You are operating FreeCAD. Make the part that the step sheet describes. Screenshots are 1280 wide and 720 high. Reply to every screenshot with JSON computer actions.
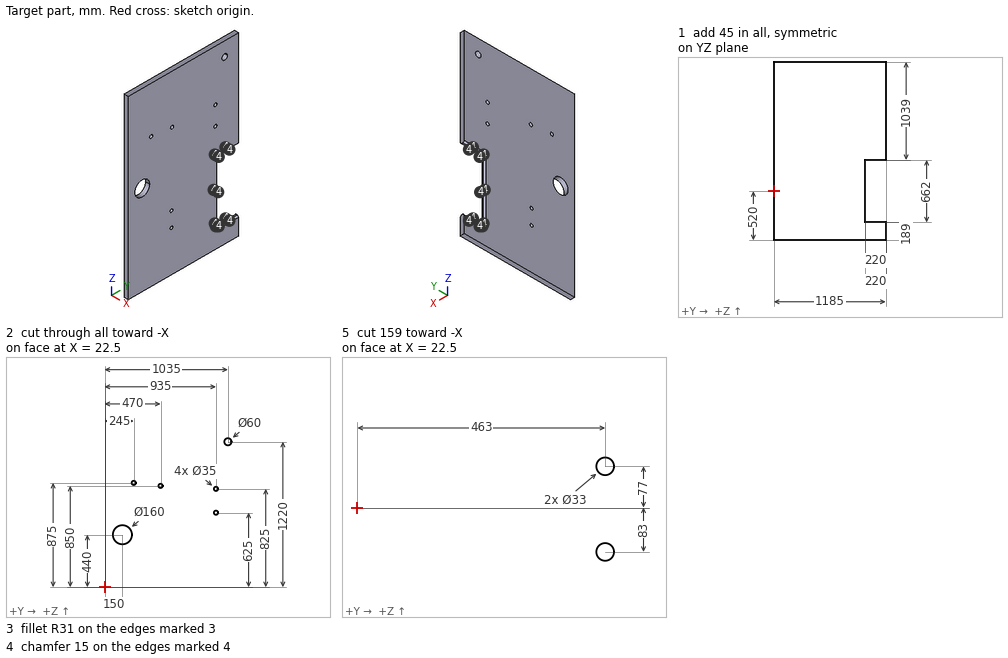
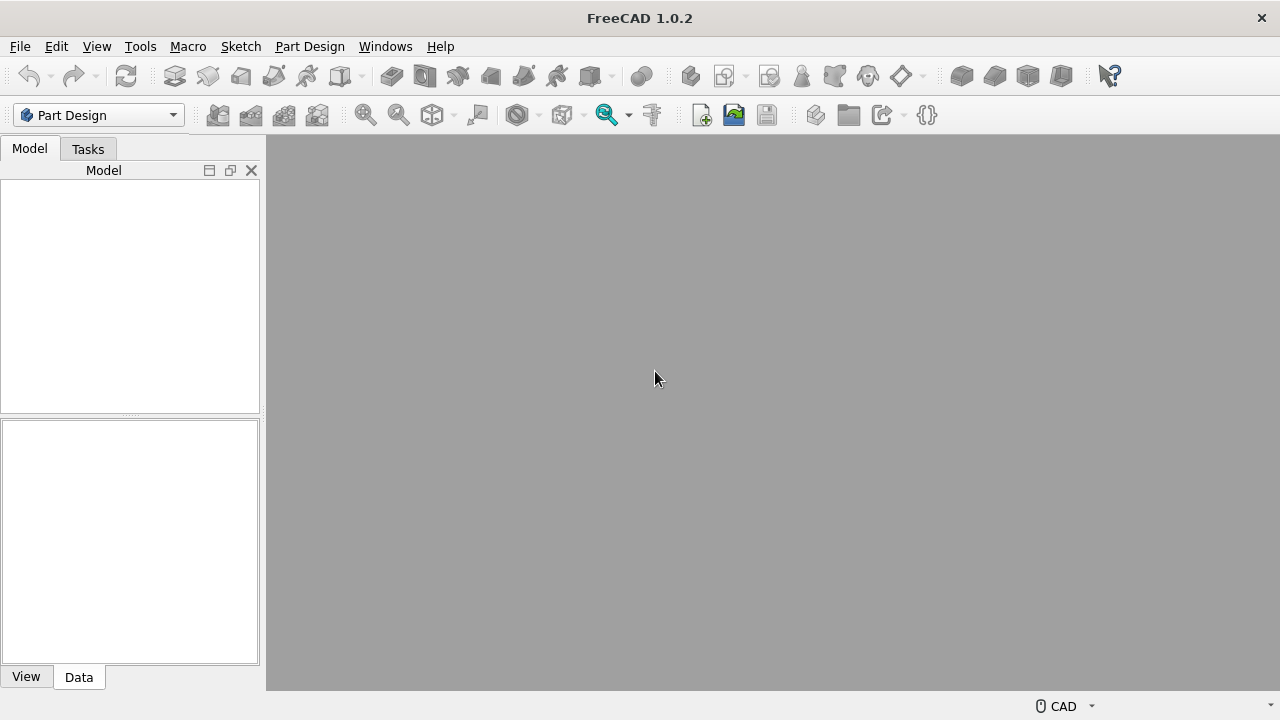
{"action": "left_click", "coordinate": [701, 116]}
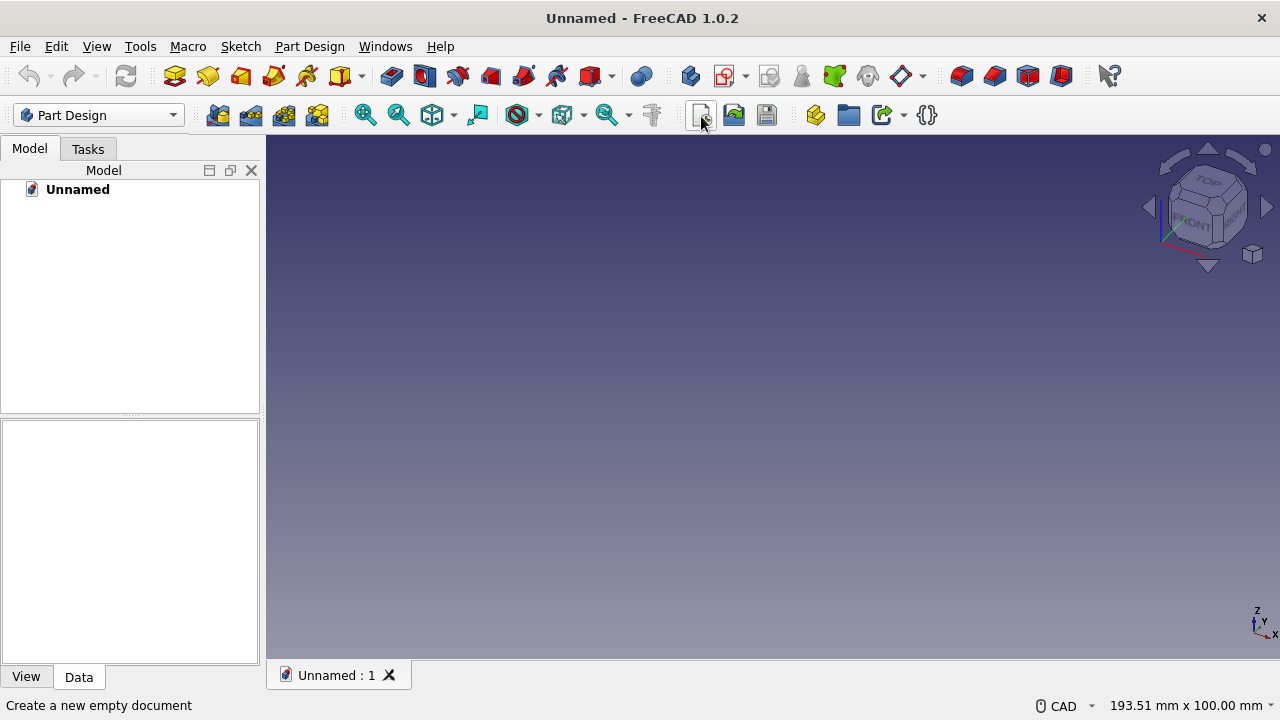
{"action": "left_click", "coordinate": [724, 76]}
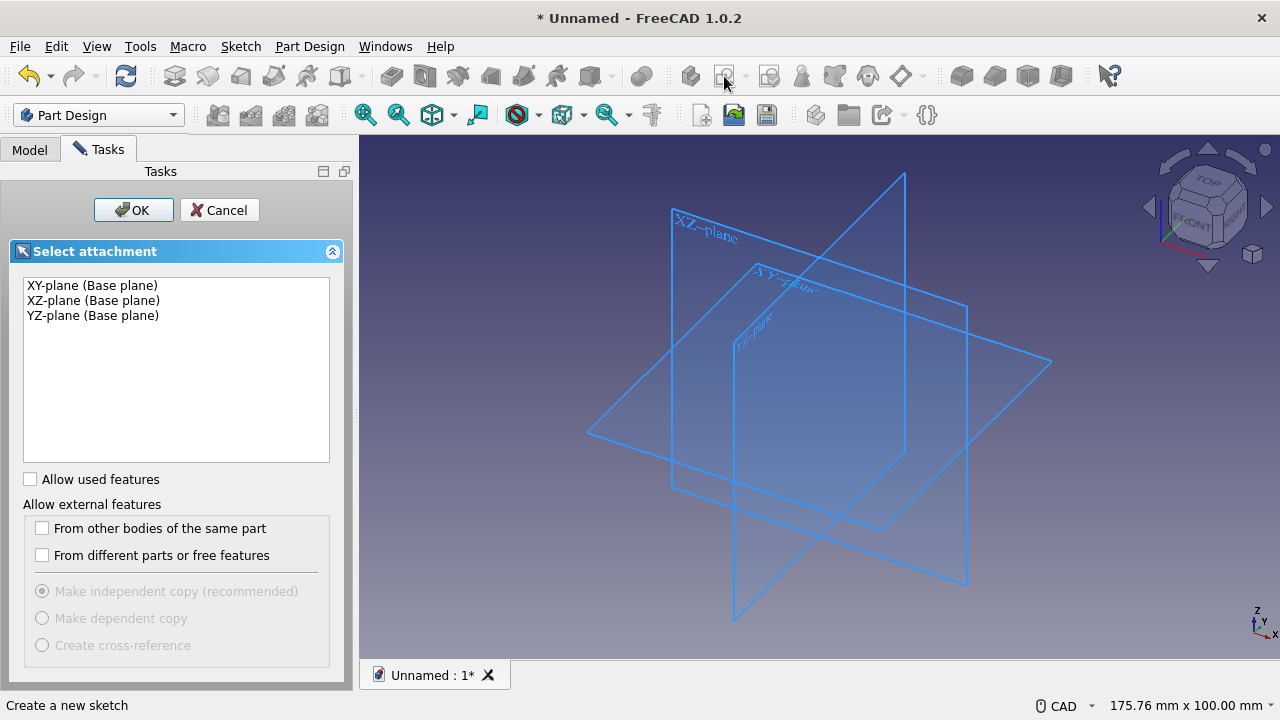
{"action": "left_click", "coordinate": [84, 316]}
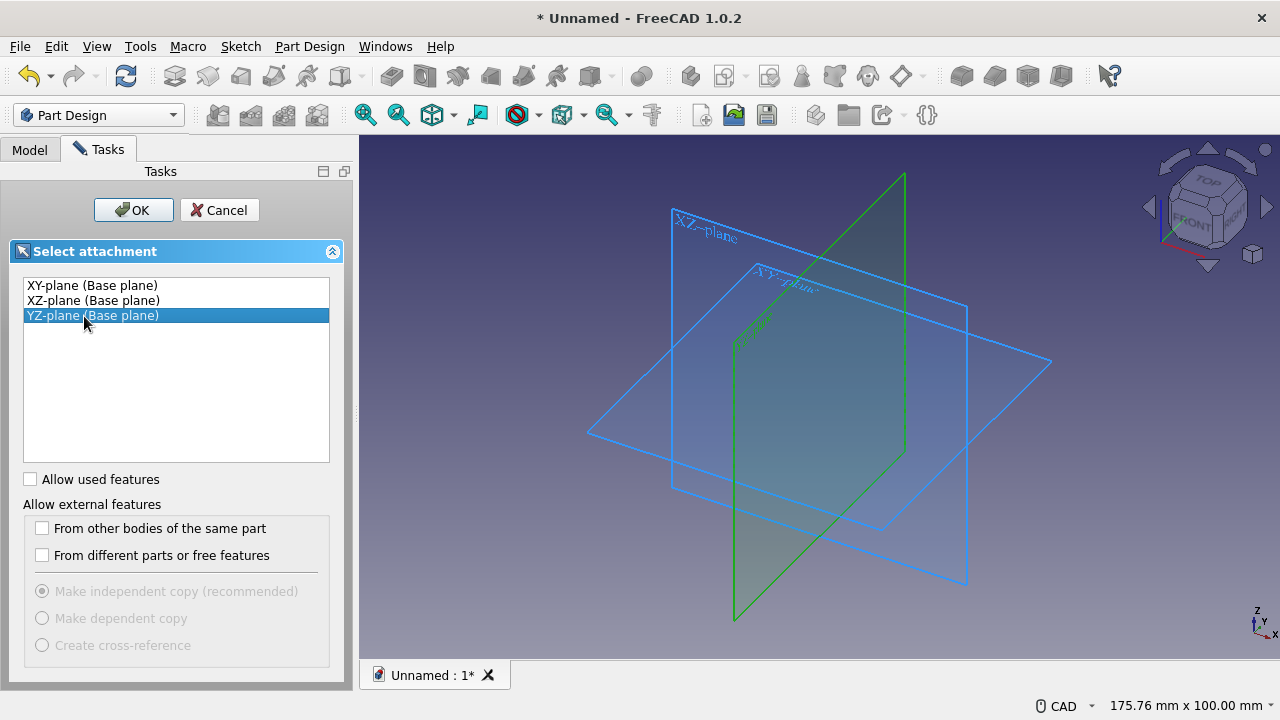
{"action": "left_click", "coordinate": [134, 210]}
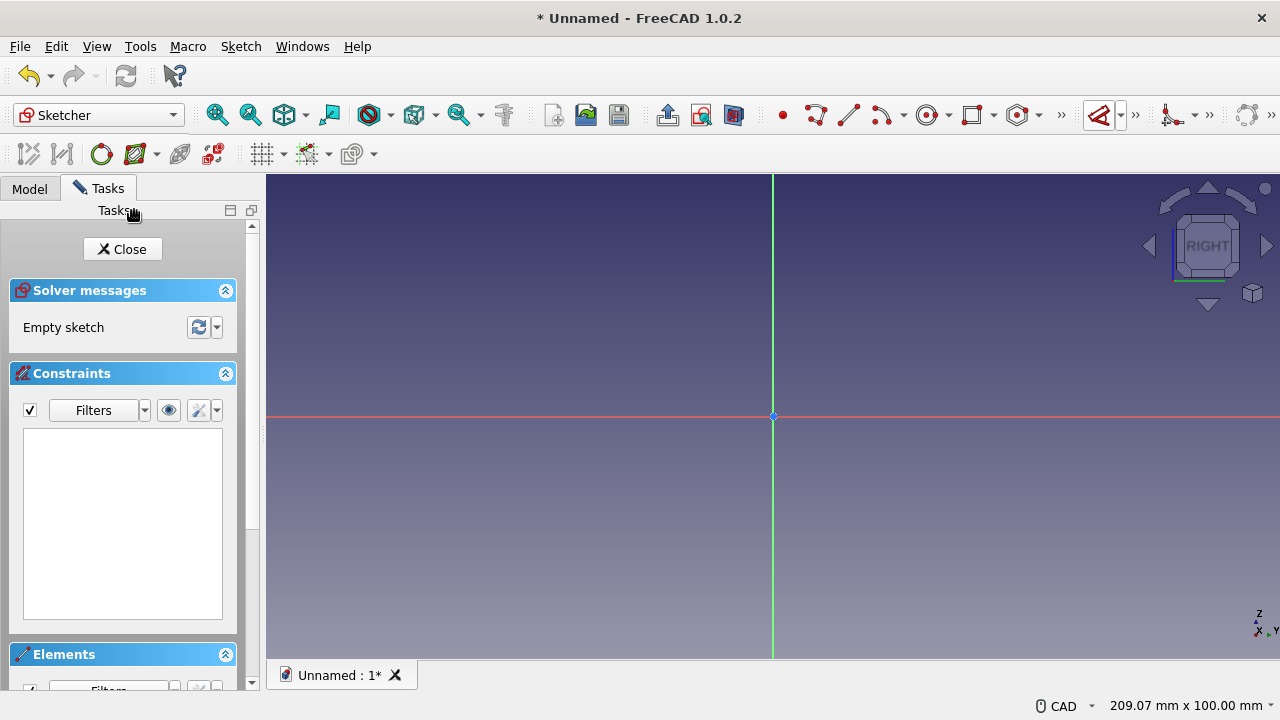
{"action": "scroll", "coordinate": [579, 504], "scroll_direction": "down", "scroll_amount": 16}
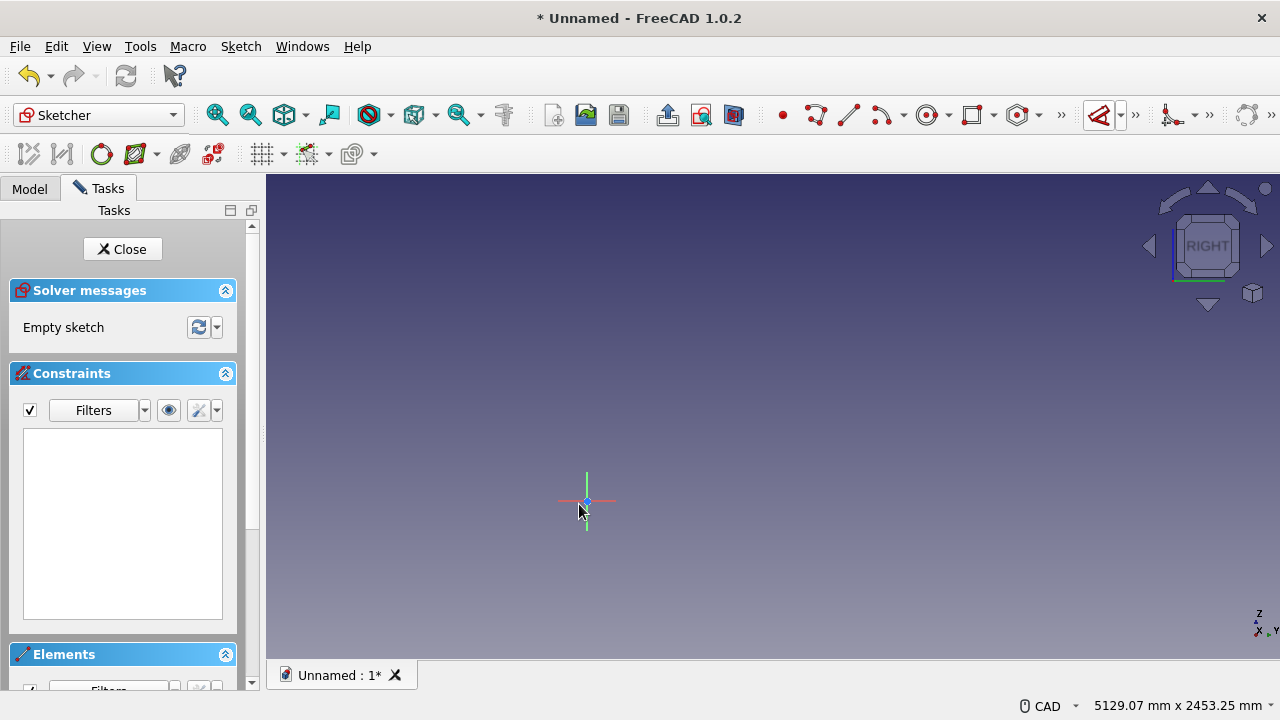
{"action": "left_click", "coordinate": [816, 116]}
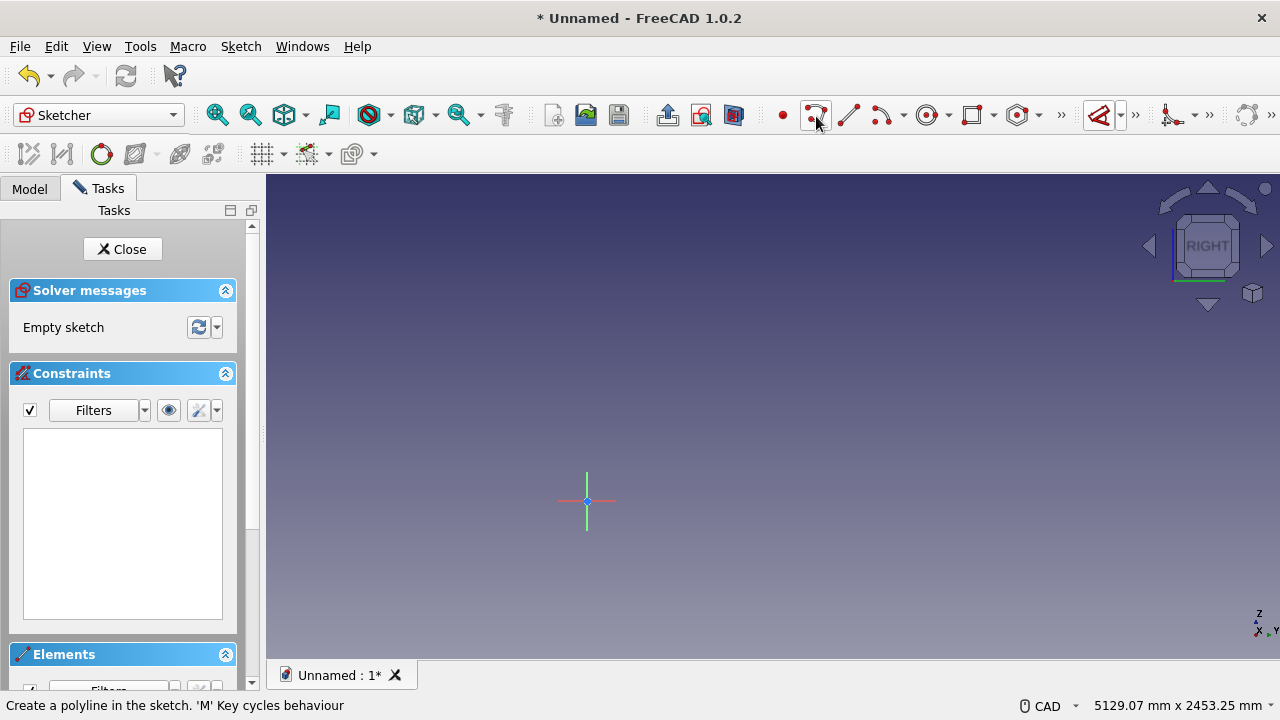
{"action": "left_click", "coordinate": [587, 604]}
{"action": "left_click", "coordinate": [821, 604]}
{"action": "left_click", "coordinate": [821, 567]}
{"action": "left_click", "coordinate": [778, 567]}
{"action": "left_click", "coordinate": [778, 436]}
{"action": "left_click", "coordinate": [821, 436]}
{"action": "left_click", "coordinate": [821, 230]}
{"action": "left_click", "coordinate": [596, 230]}
{"action": "left_click", "coordinate": [587, 605]}
{"action": "key", "text": "Escape"}
{"action": "key", "text": "Escape"}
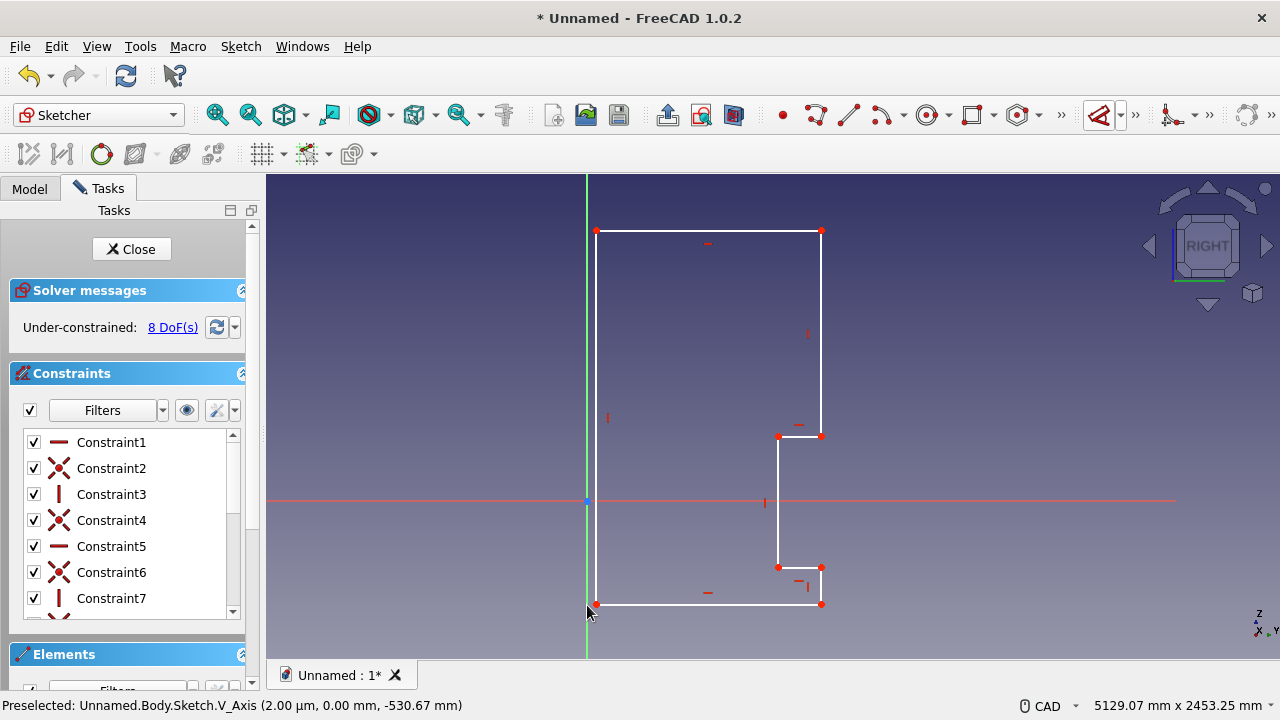
{"action": "left_click", "coordinate": [596, 605]}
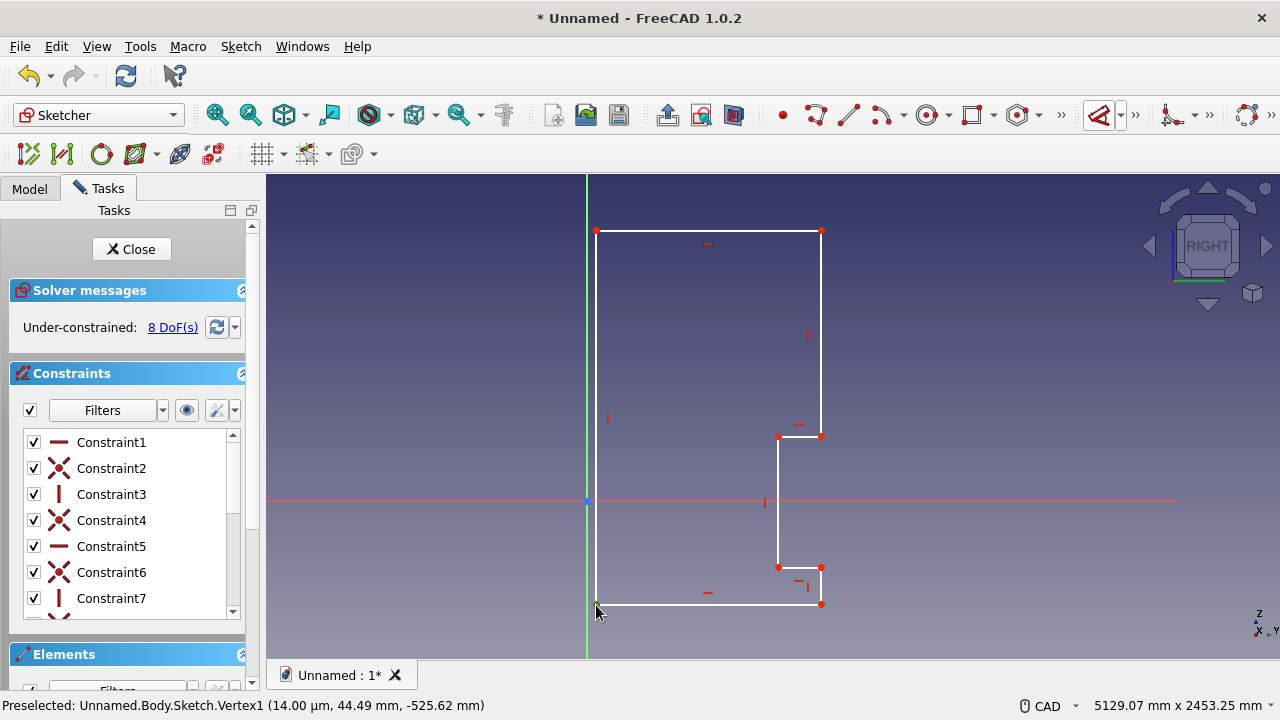
{"action": "left_click", "coordinate": [587, 600]}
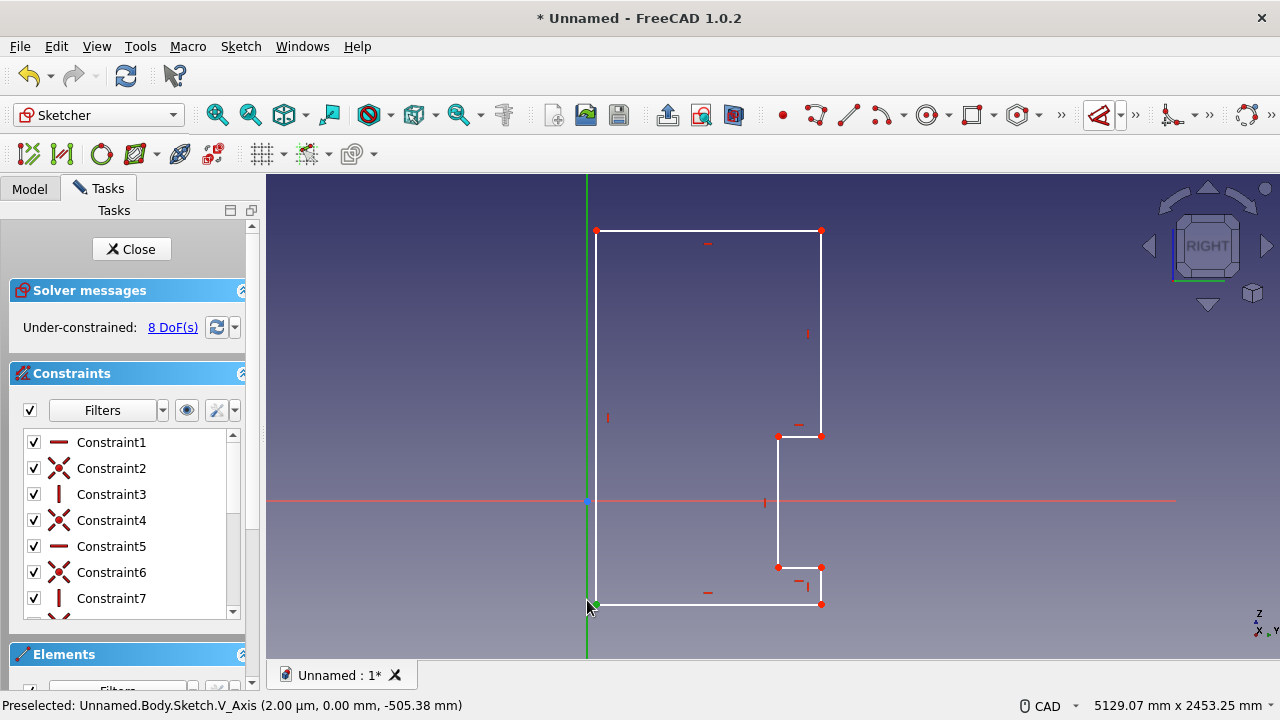
{"action": "key", "text": "c"}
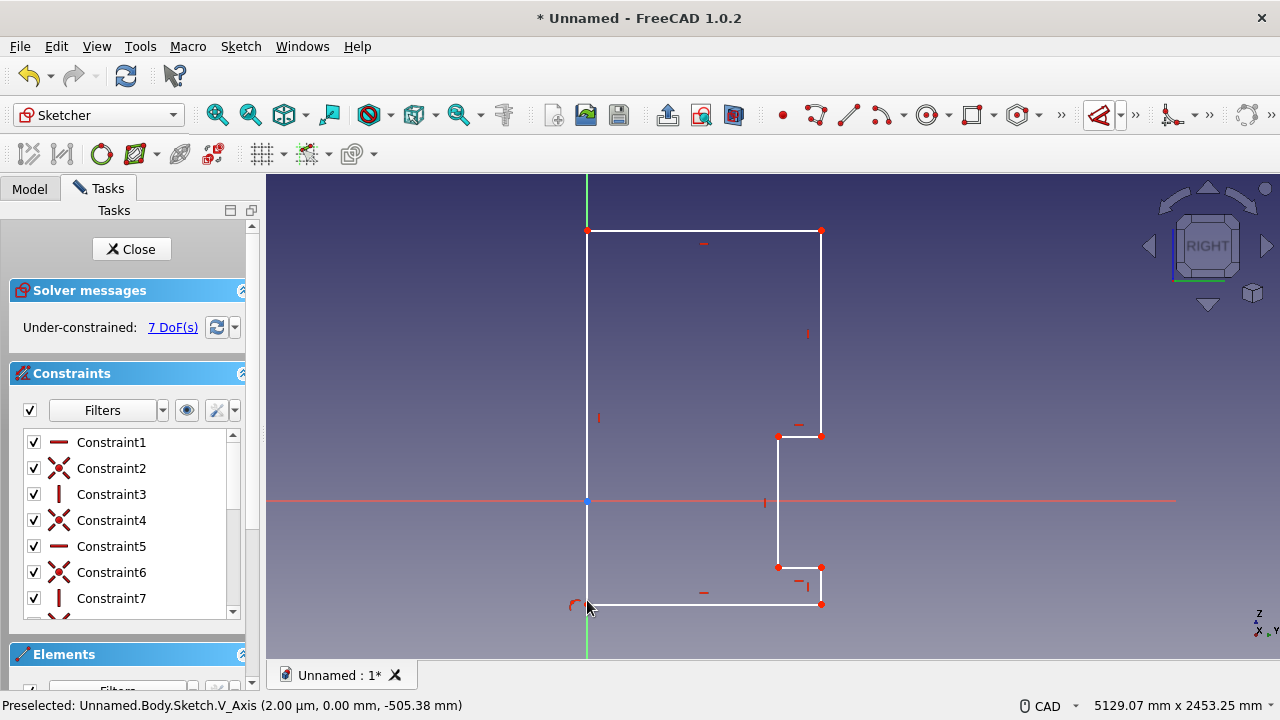
{"action": "scroll", "coordinate": [821, 594], "scroll_direction": "up", "scroll_amount": 2}